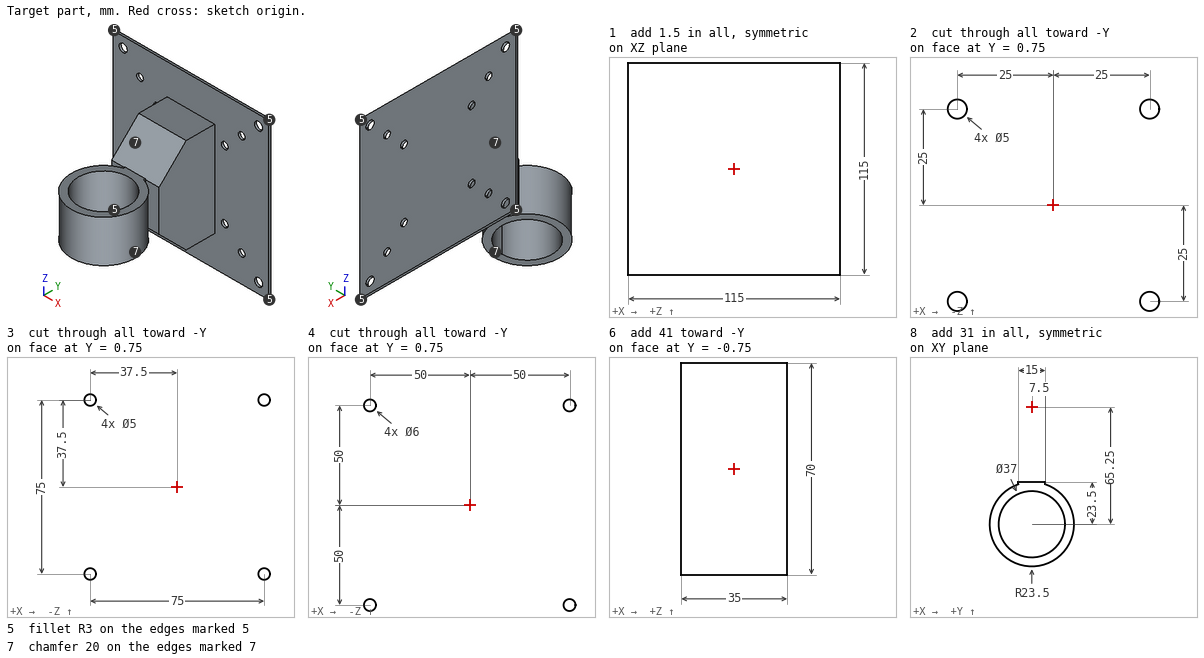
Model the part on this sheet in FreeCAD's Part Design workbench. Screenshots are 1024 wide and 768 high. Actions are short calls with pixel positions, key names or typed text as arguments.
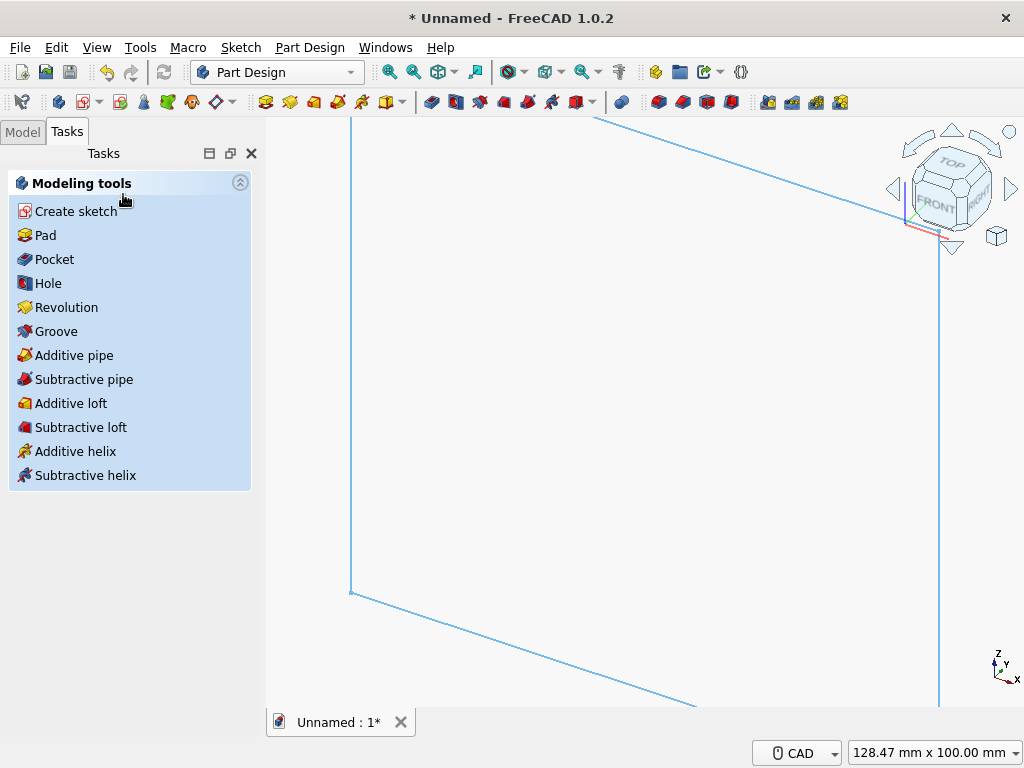
click(266, 102)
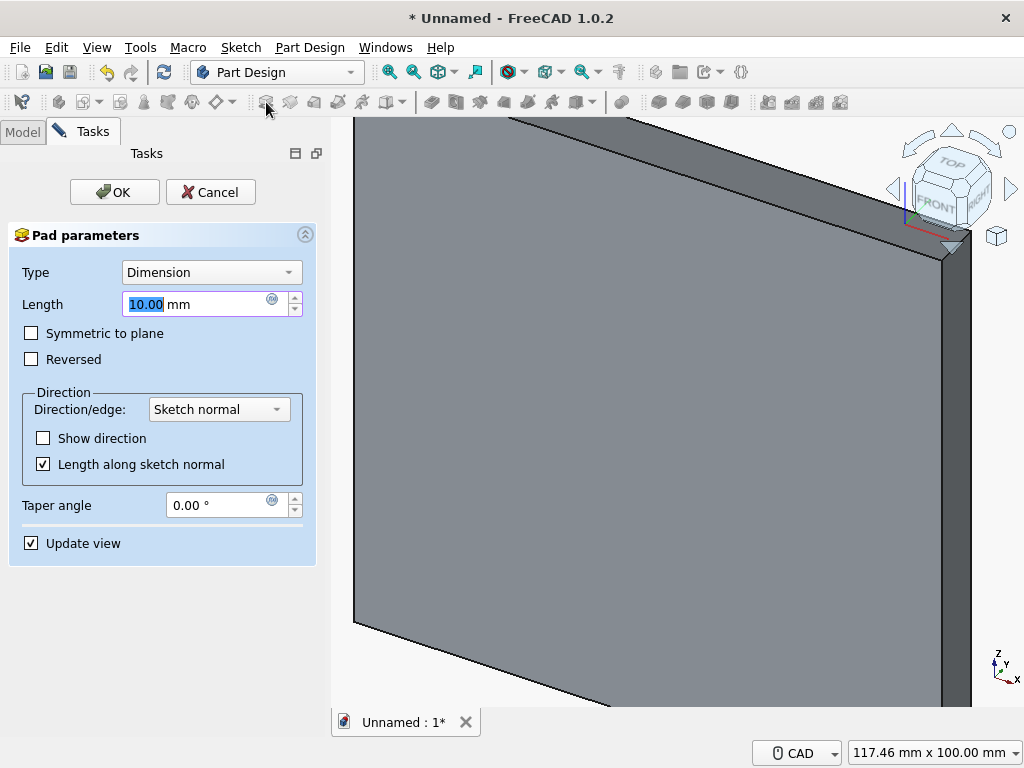
text(1.5)
key(Tab)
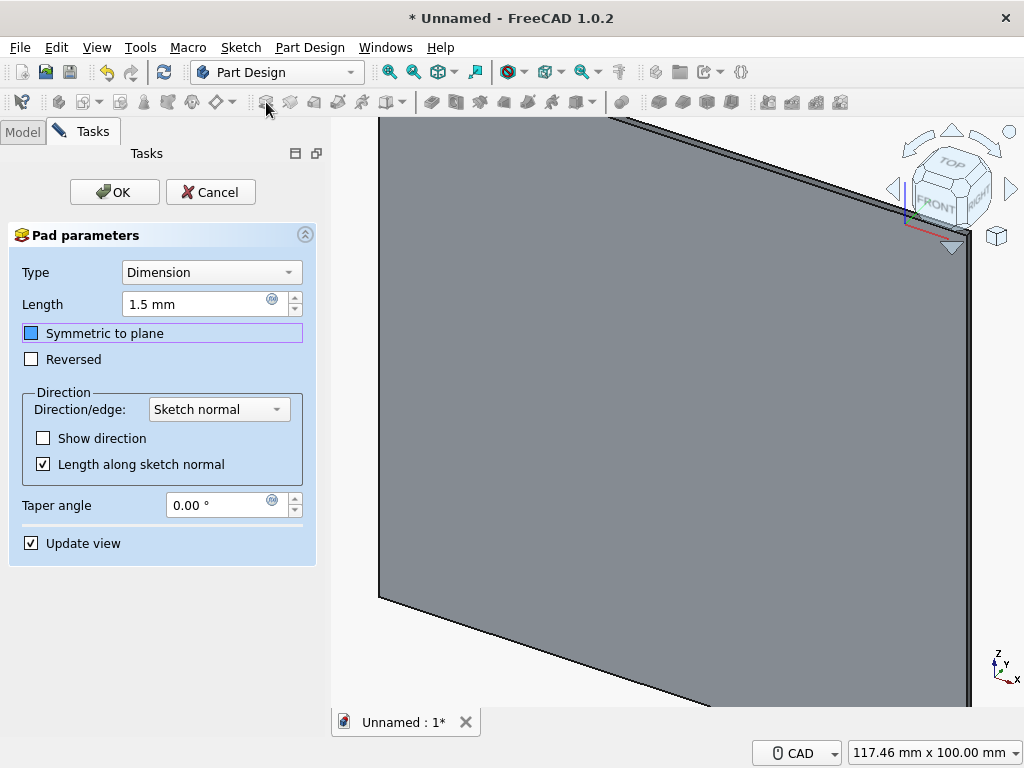
click(30, 333)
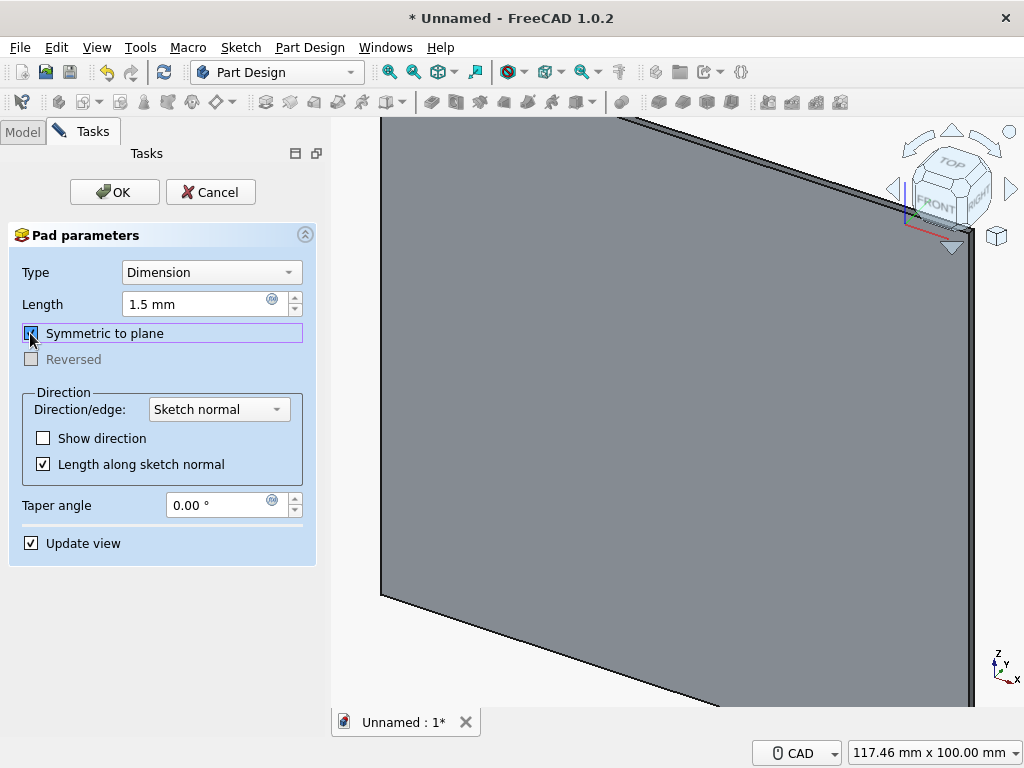
click(115, 192)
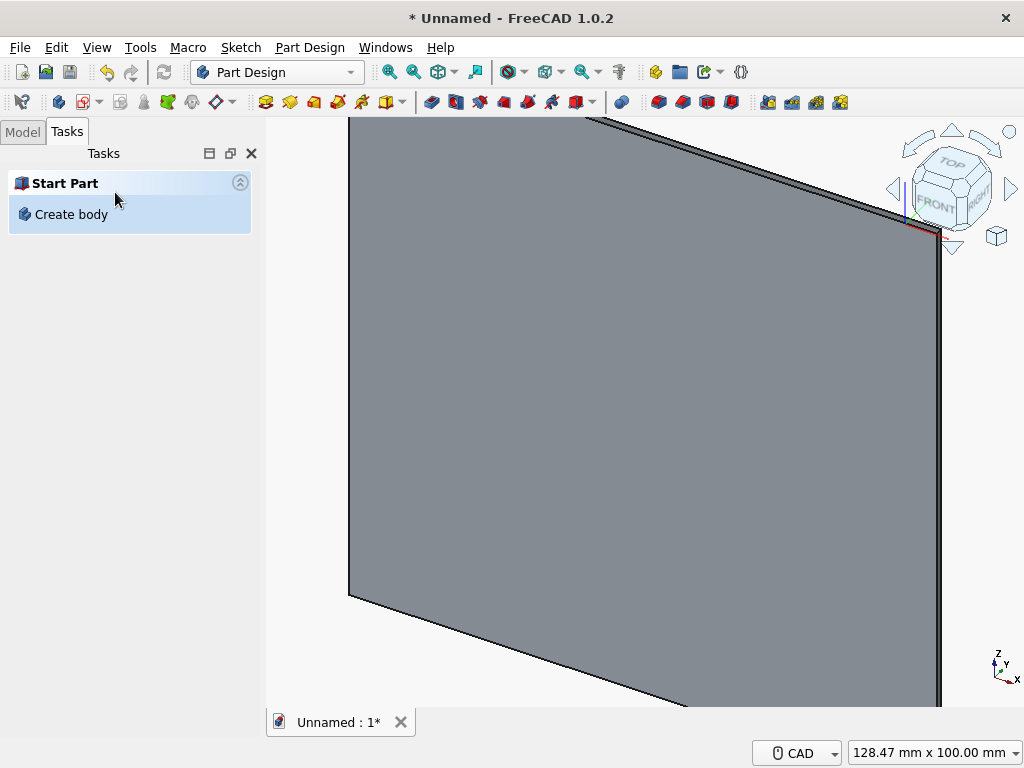
click(390, 72)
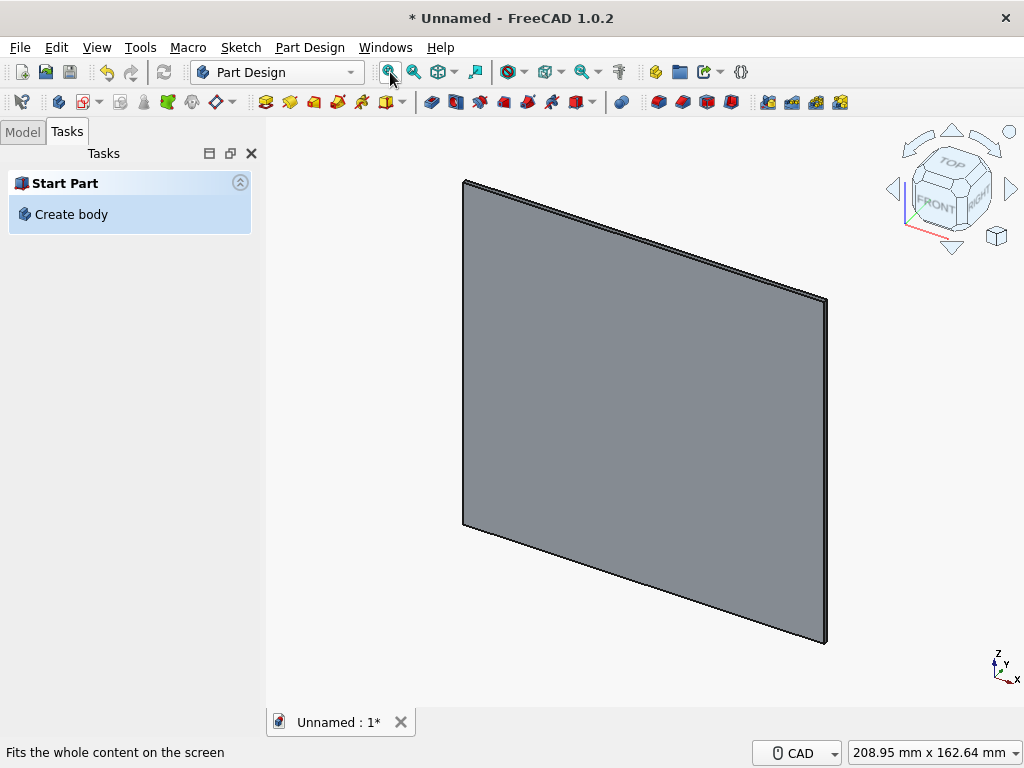
key(4)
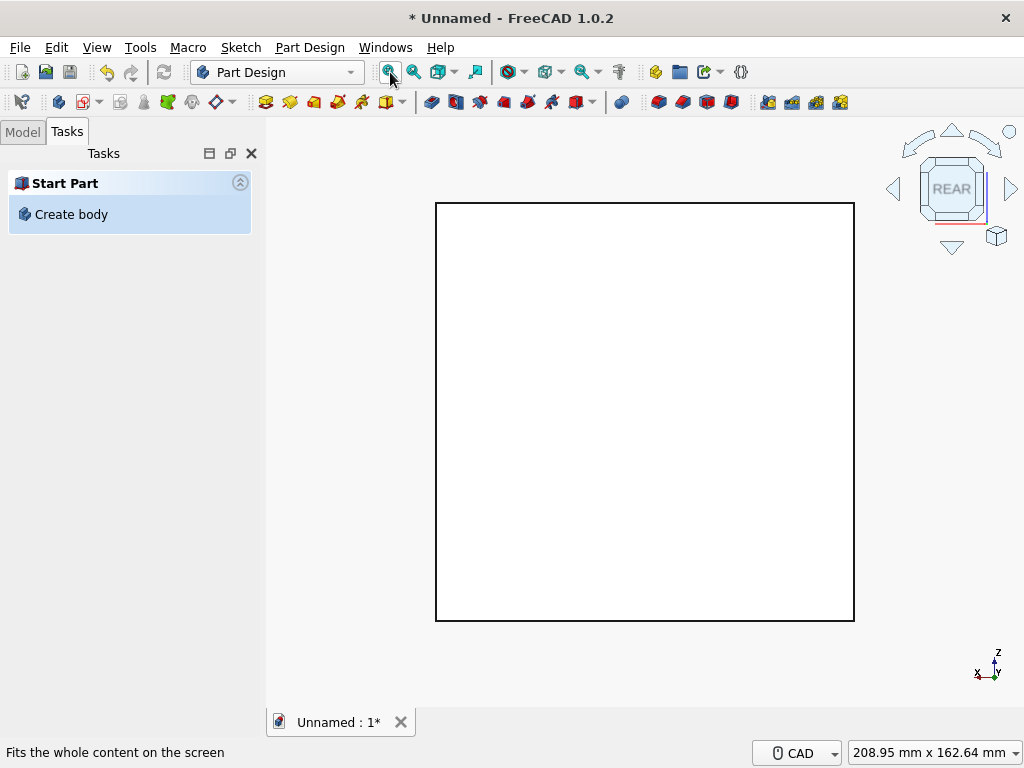
click(645, 411)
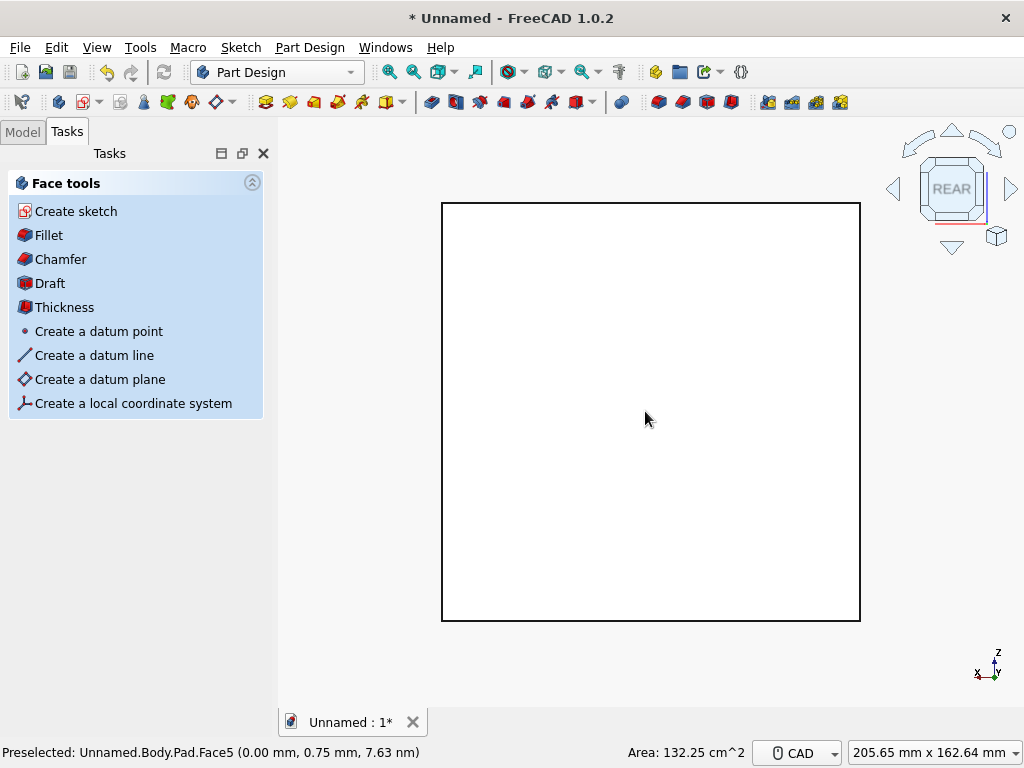
click(84, 102)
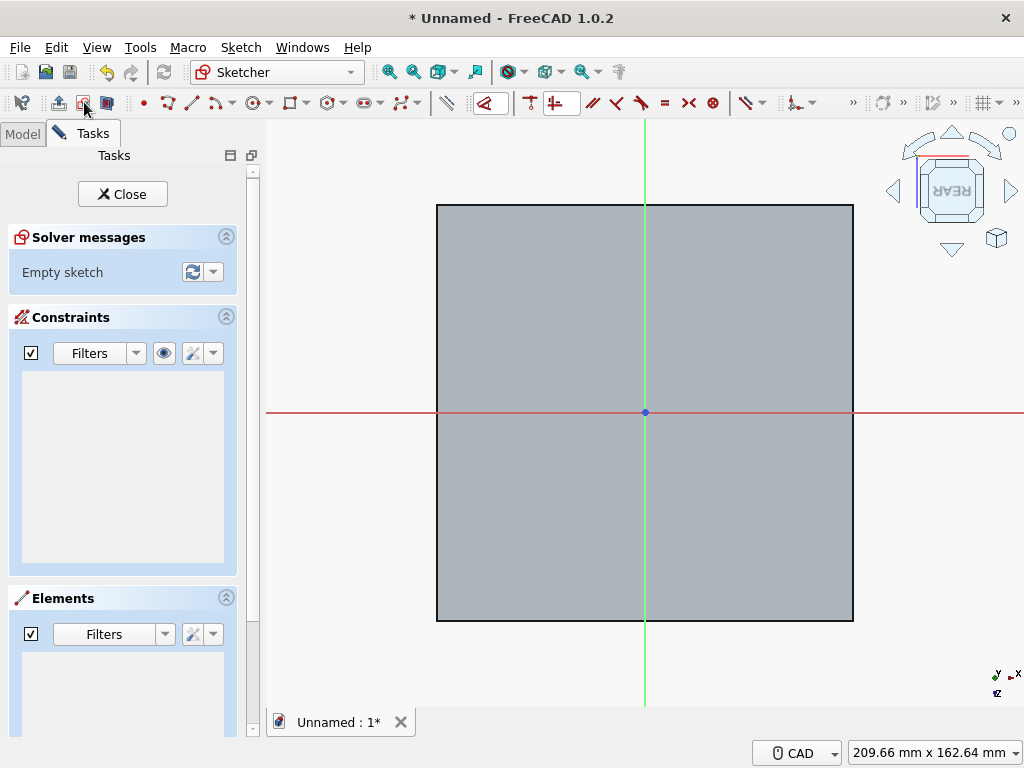
scroll(728, 413, up, 3)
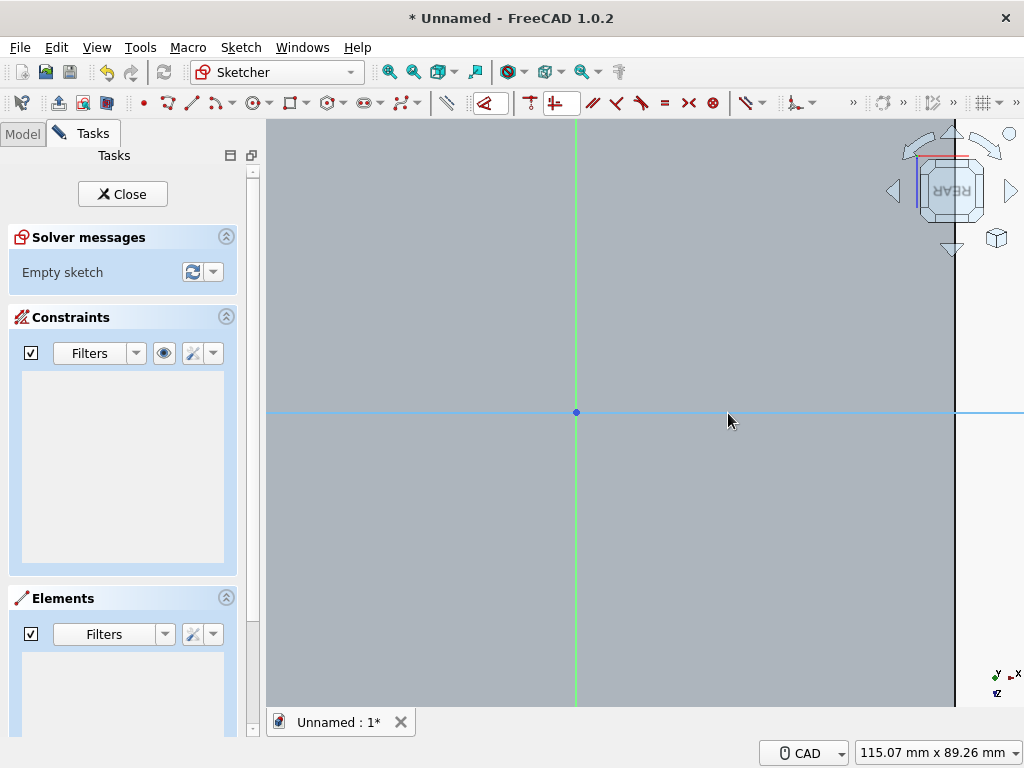
key(g)
key(c)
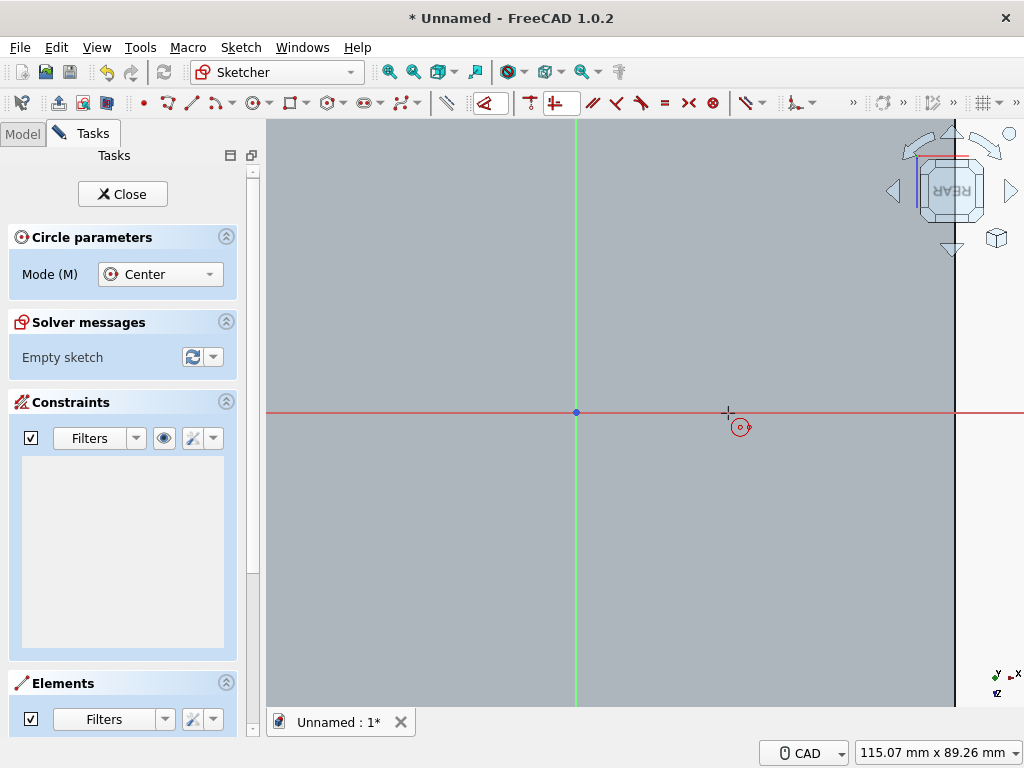
scroll(412, 248, up, 2)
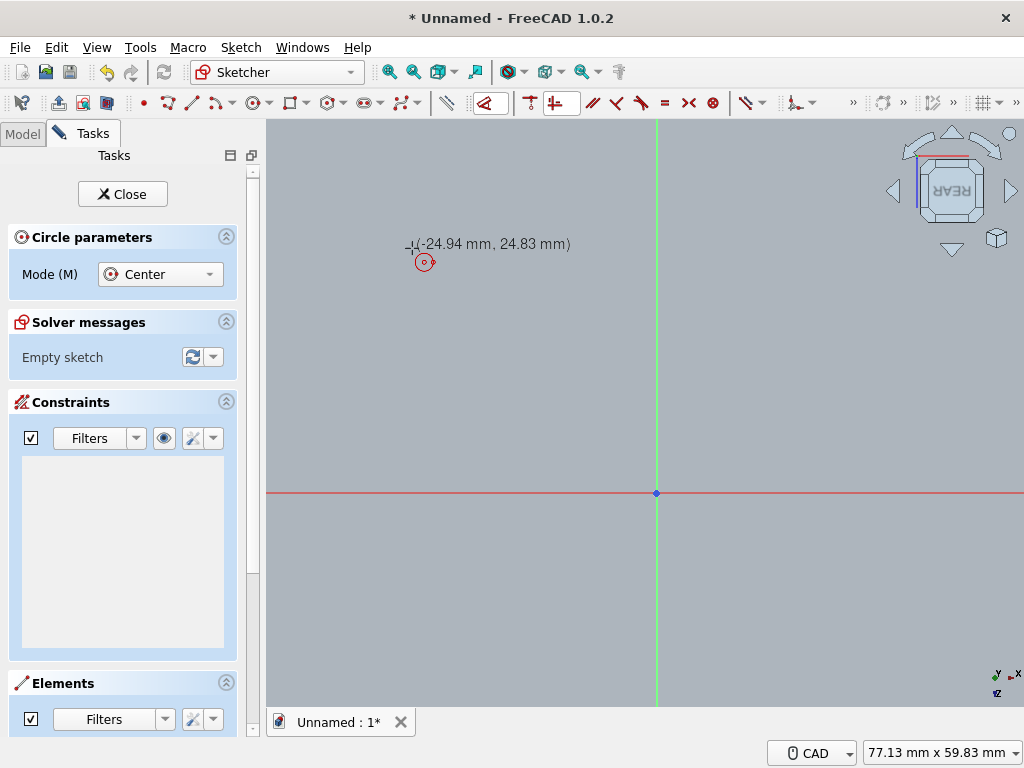
click(411, 248)
click(429, 230)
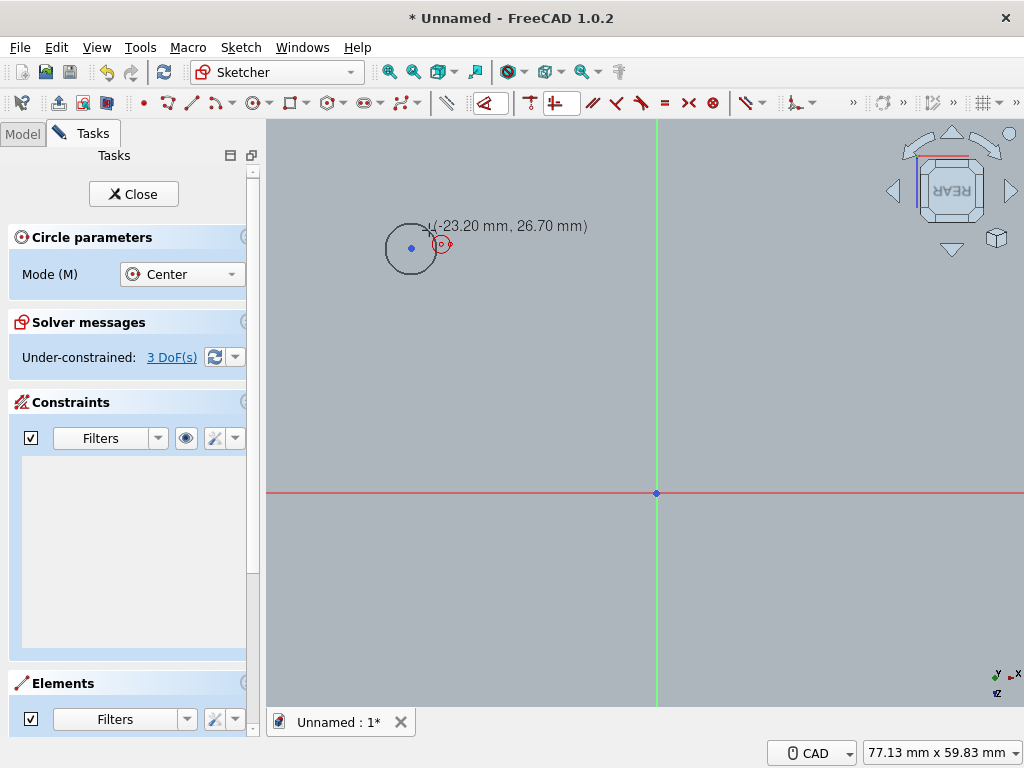
scroll(413, 249, down, 2)